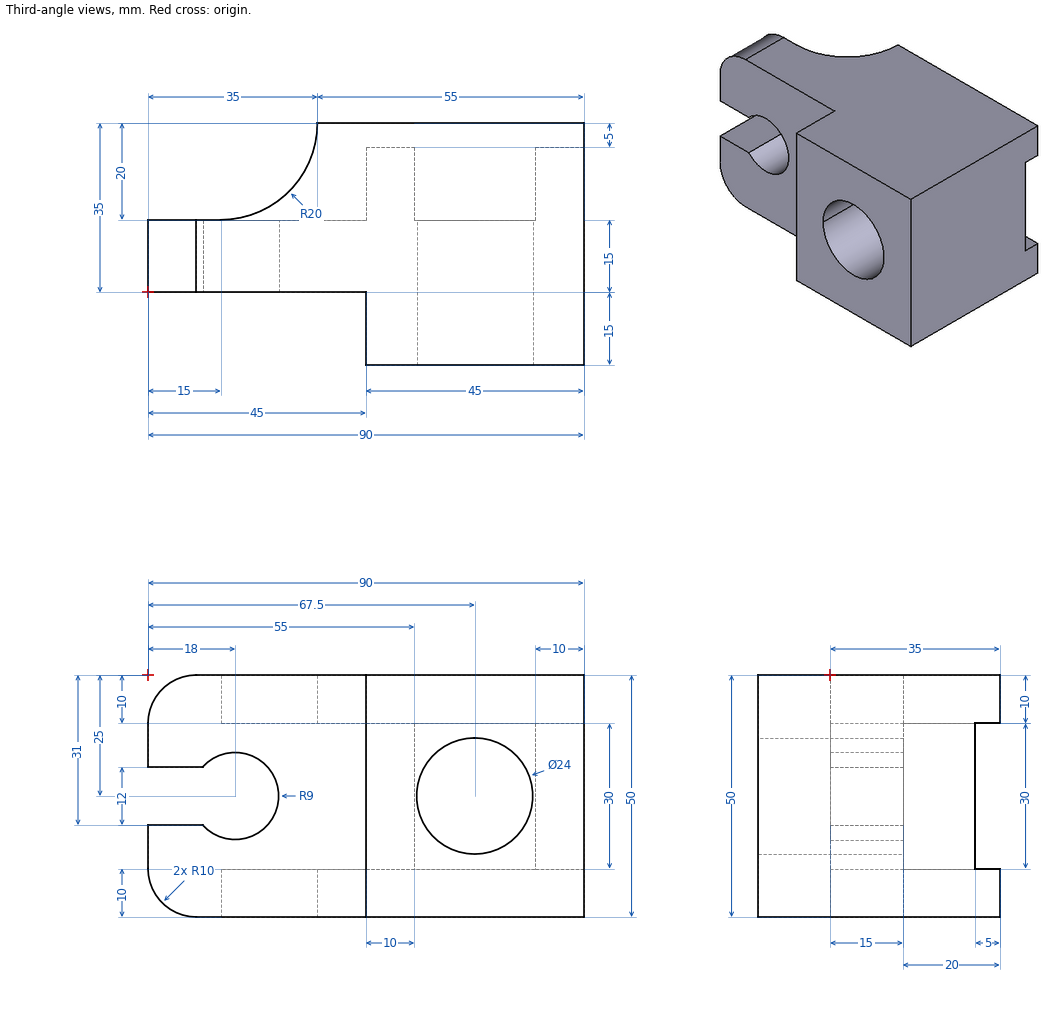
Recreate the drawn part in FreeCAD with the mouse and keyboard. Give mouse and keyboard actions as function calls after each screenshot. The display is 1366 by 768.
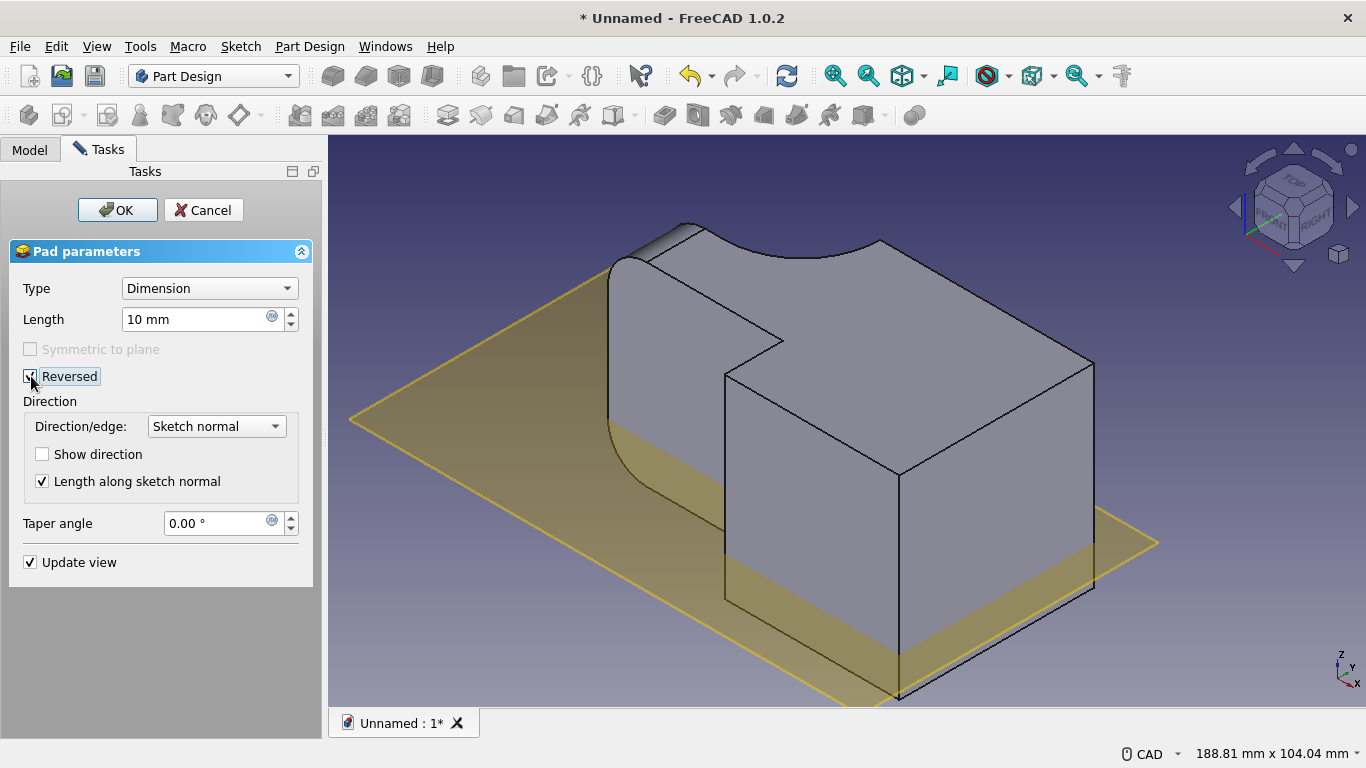
click(118, 210)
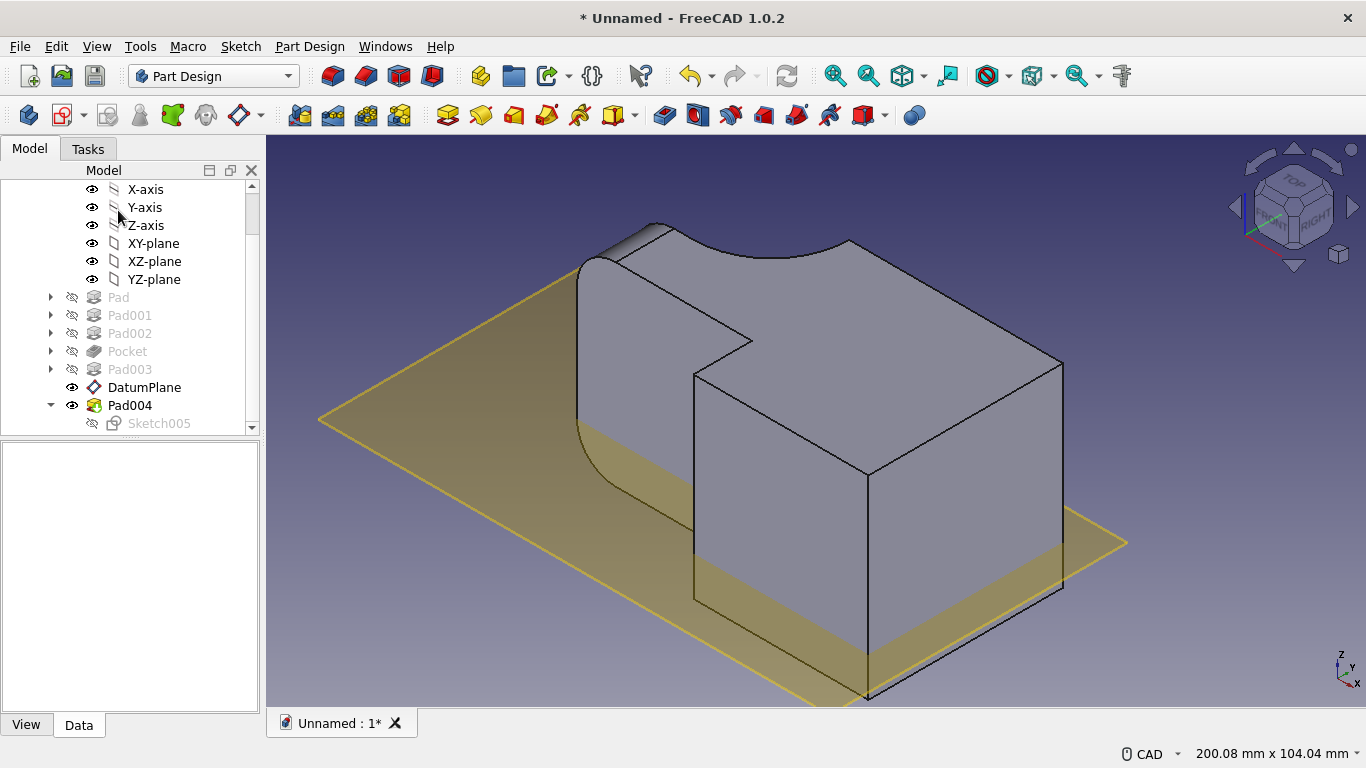
click(117, 387)
key(space)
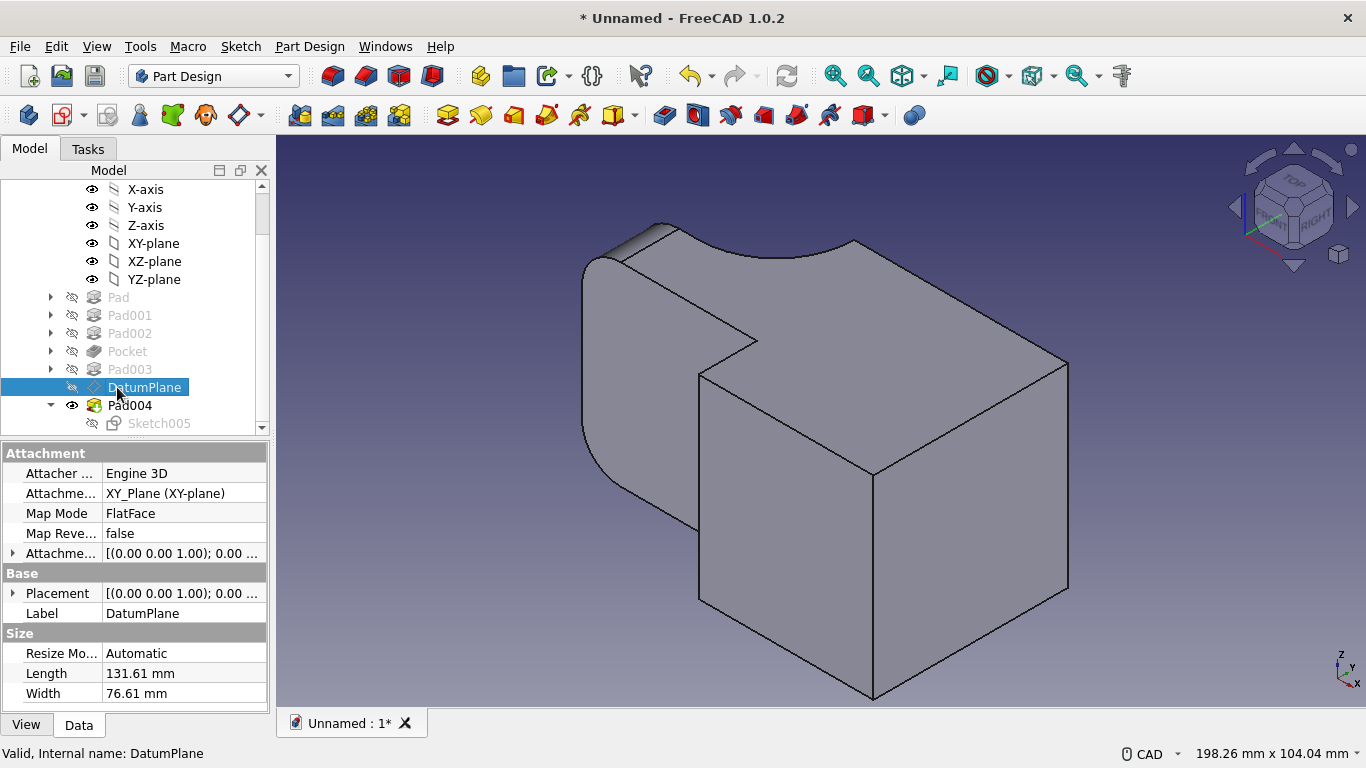
key(4)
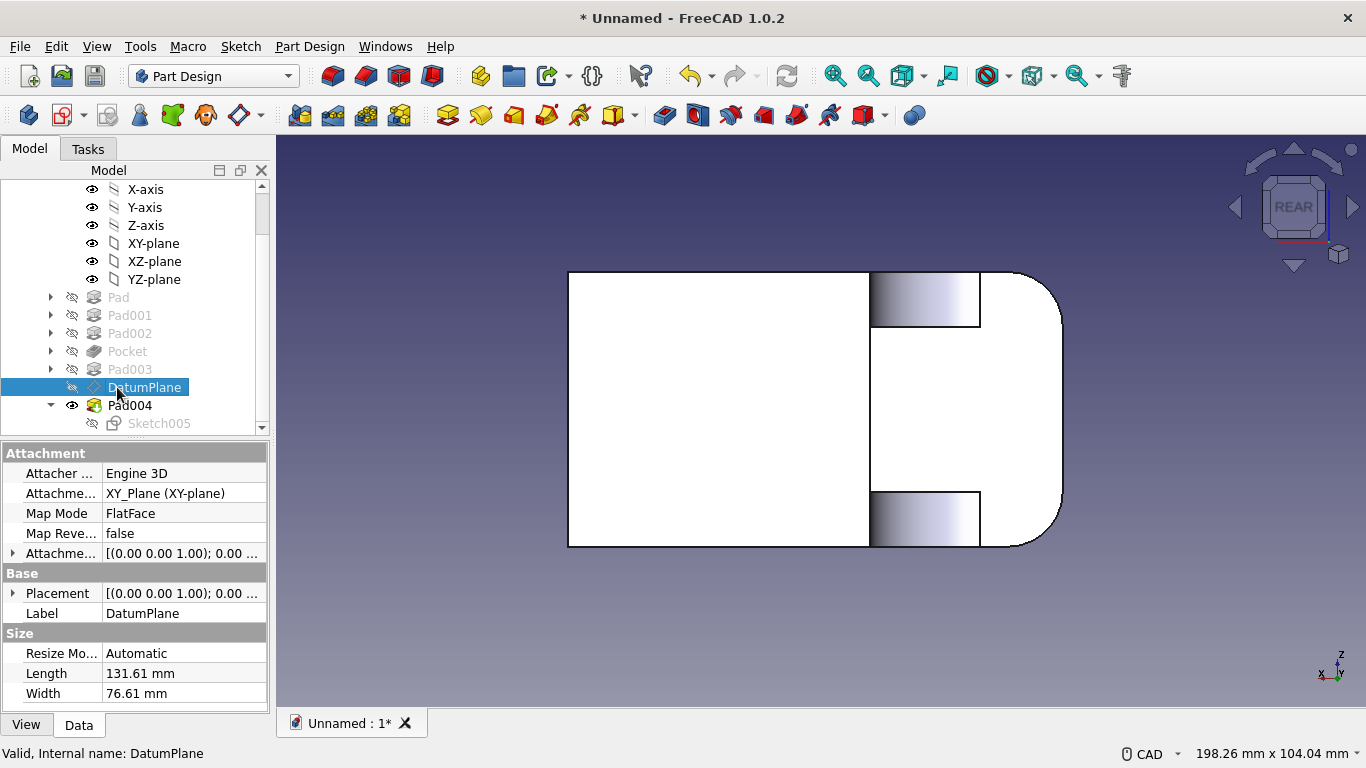
click(967, 408)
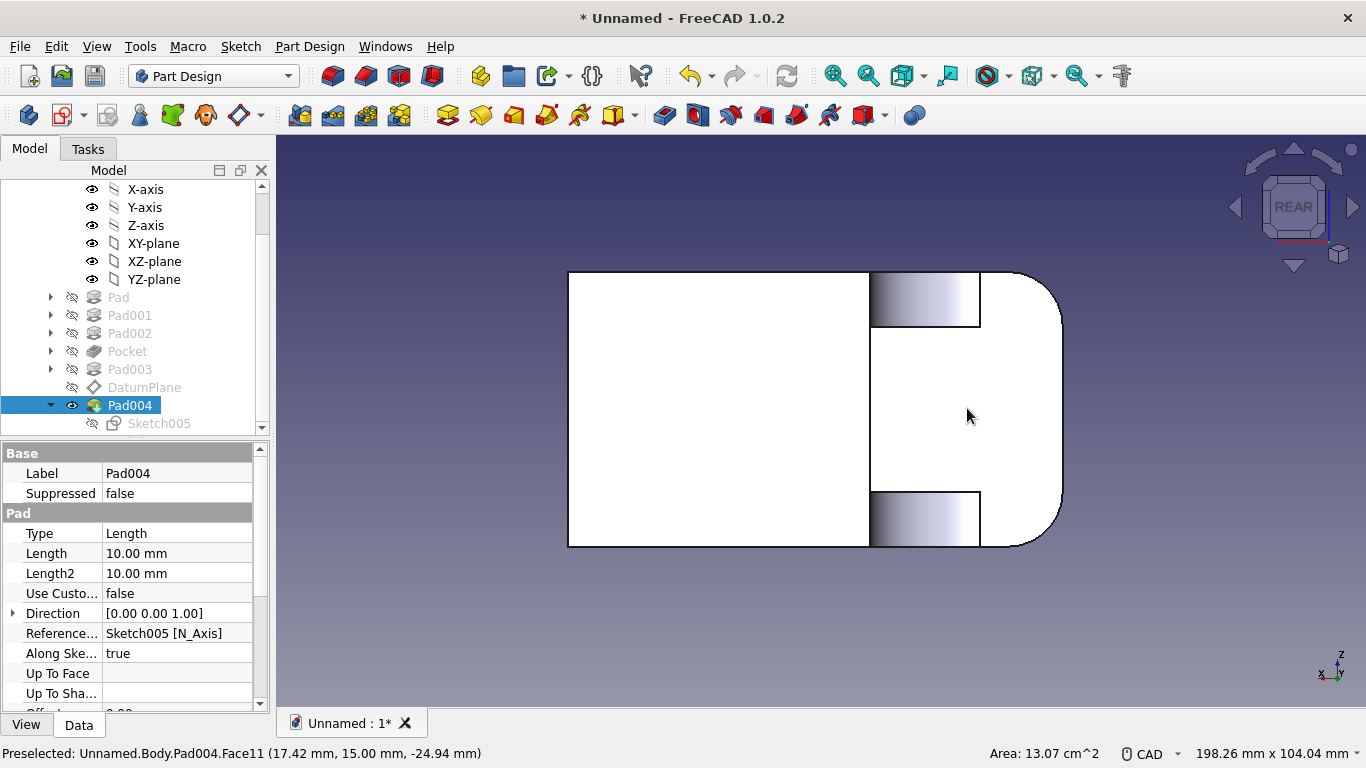
click(62, 116)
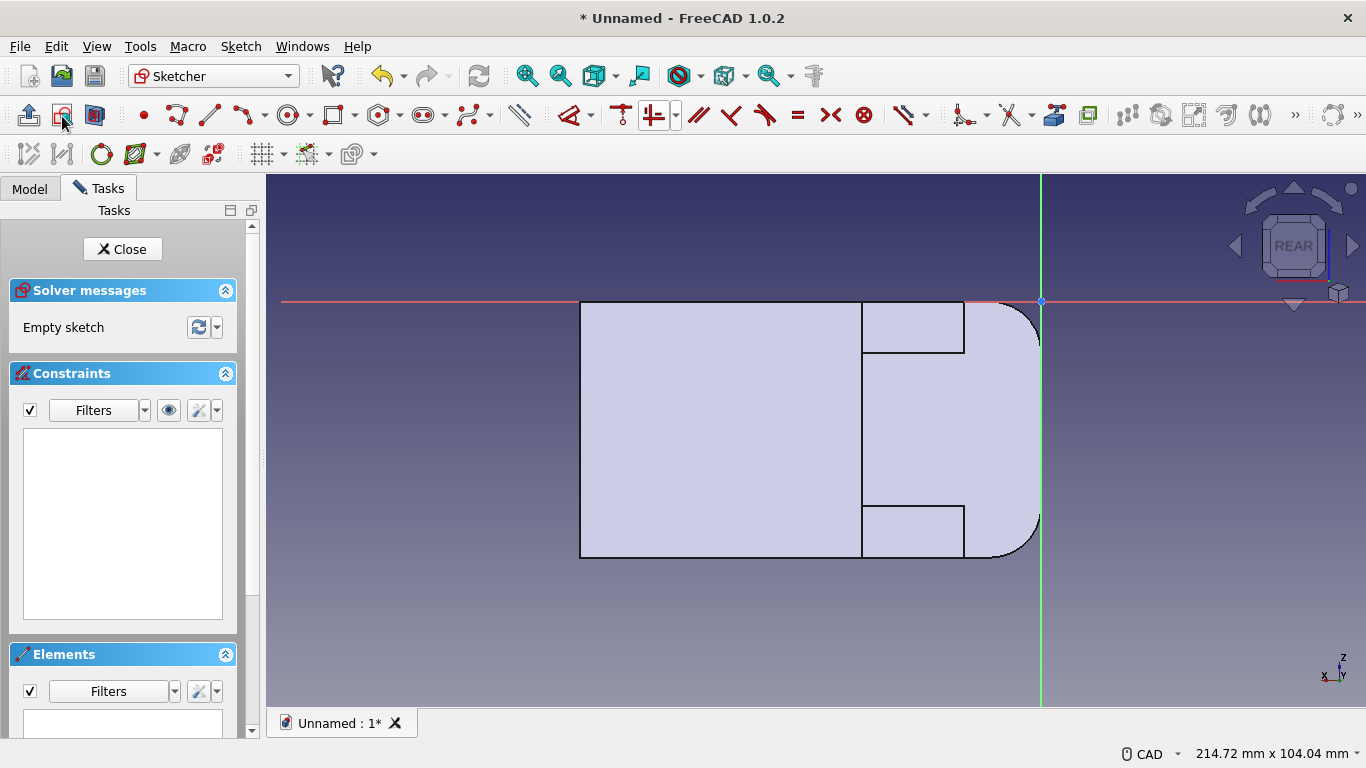
key(q)
key(s)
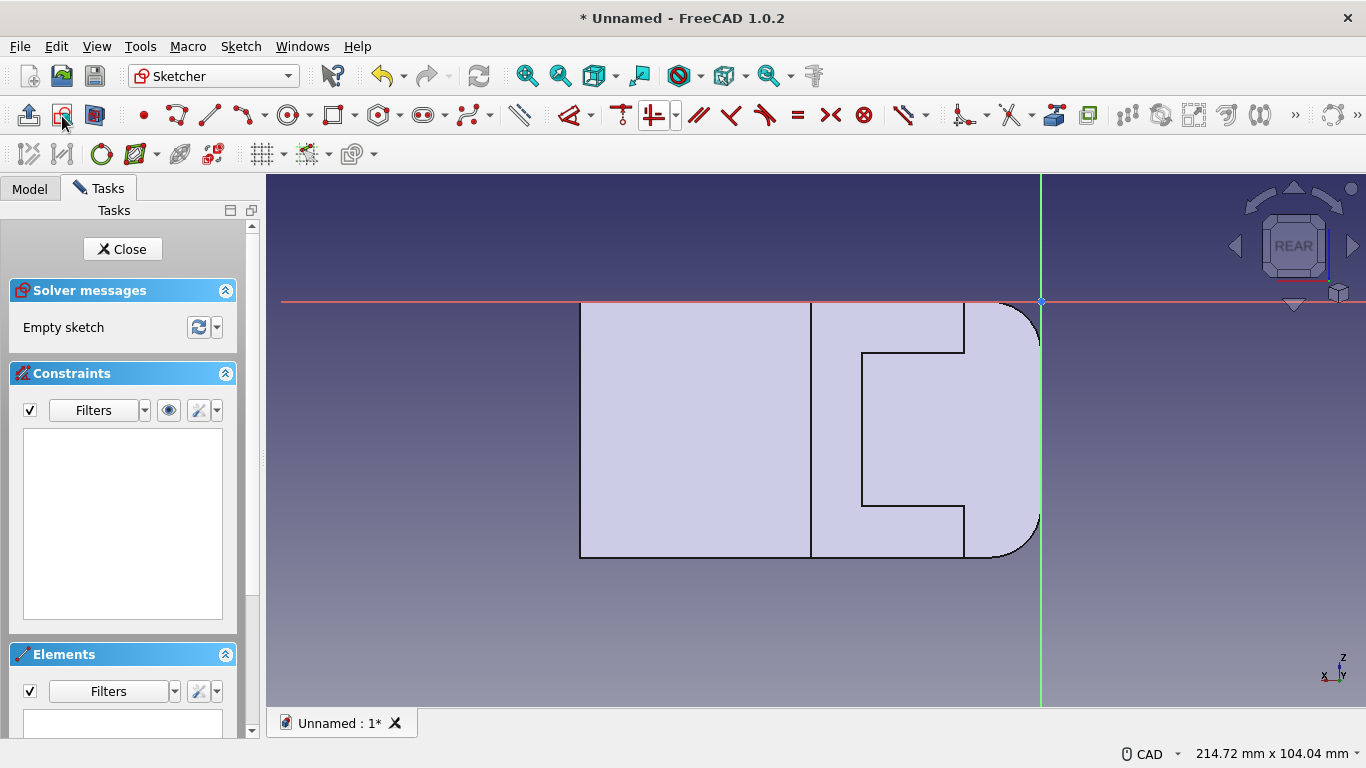
scroll(1155, 332, up, 4)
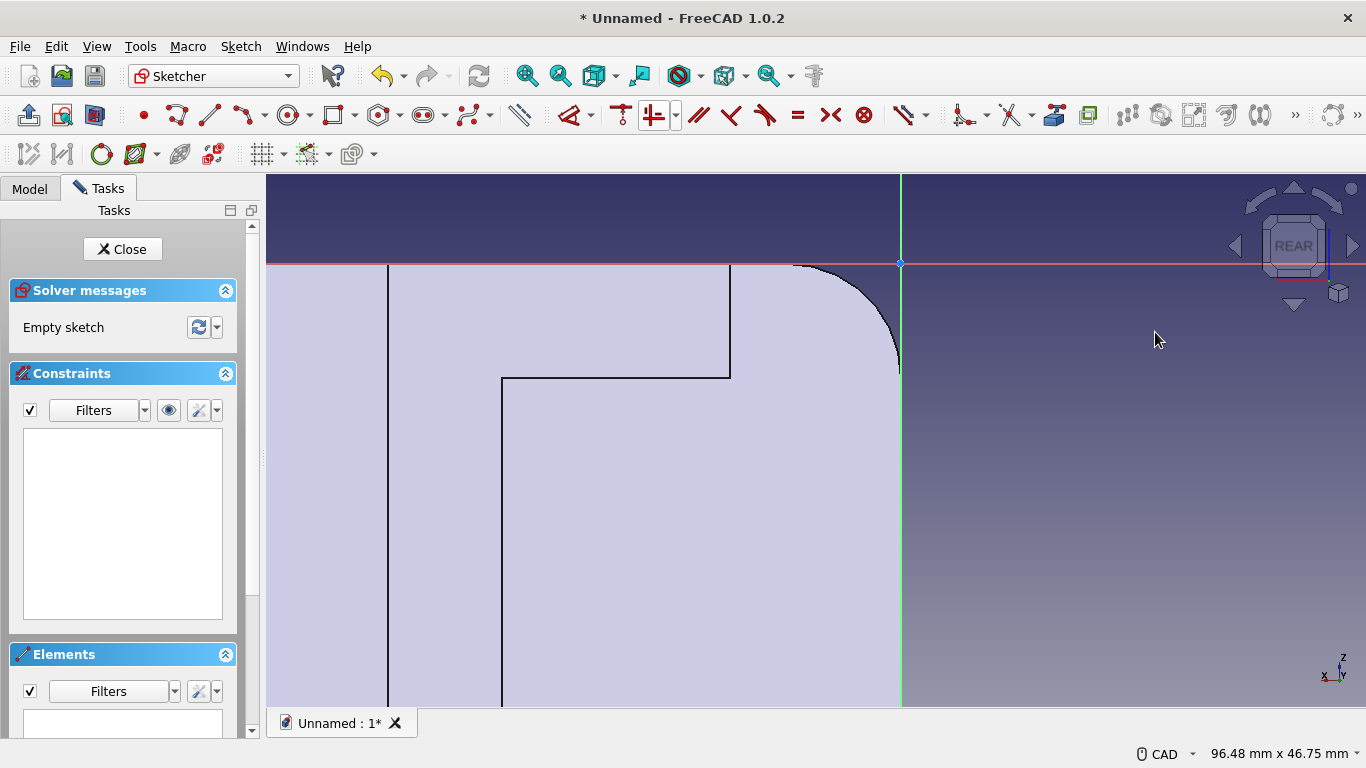
key(g)
key(m)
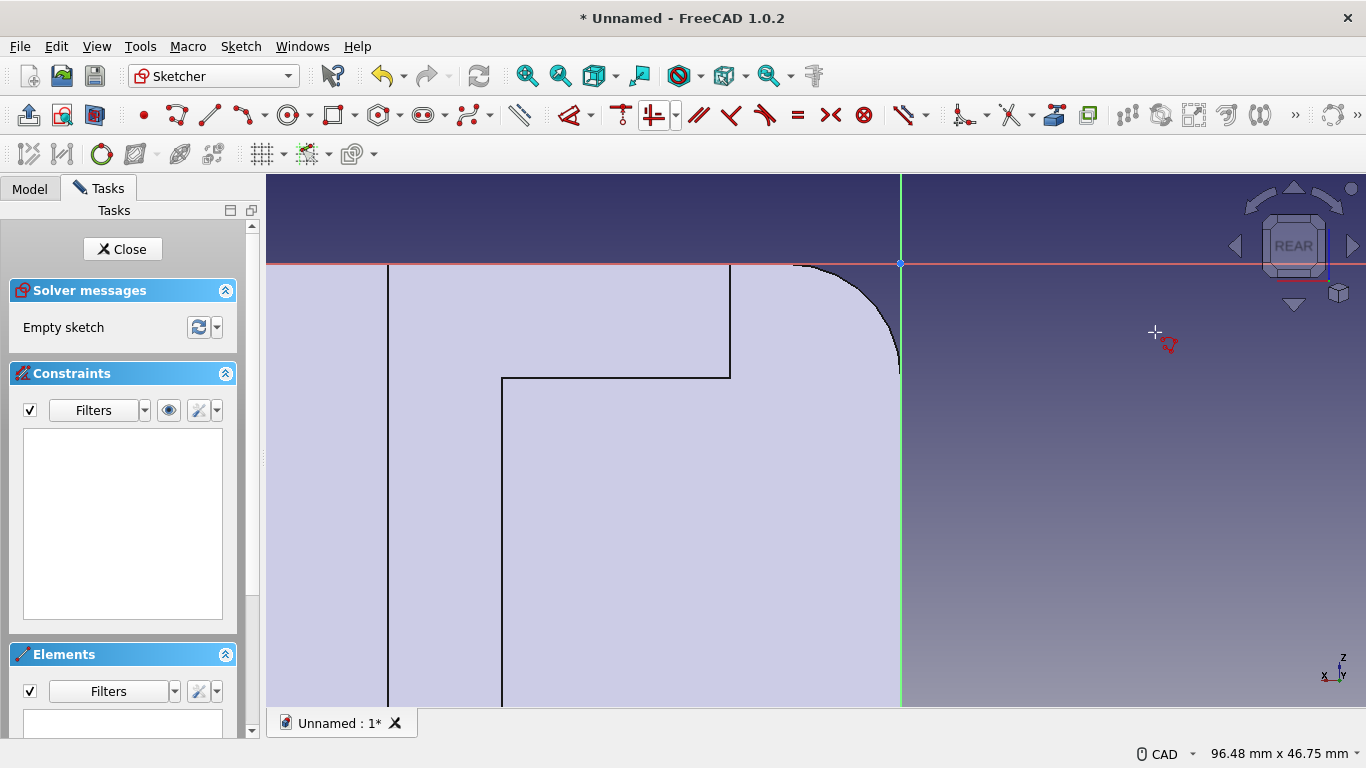
click(772, 617)
click(901, 617)
click(892, 480)
click(772, 480)
right_click(772, 480)